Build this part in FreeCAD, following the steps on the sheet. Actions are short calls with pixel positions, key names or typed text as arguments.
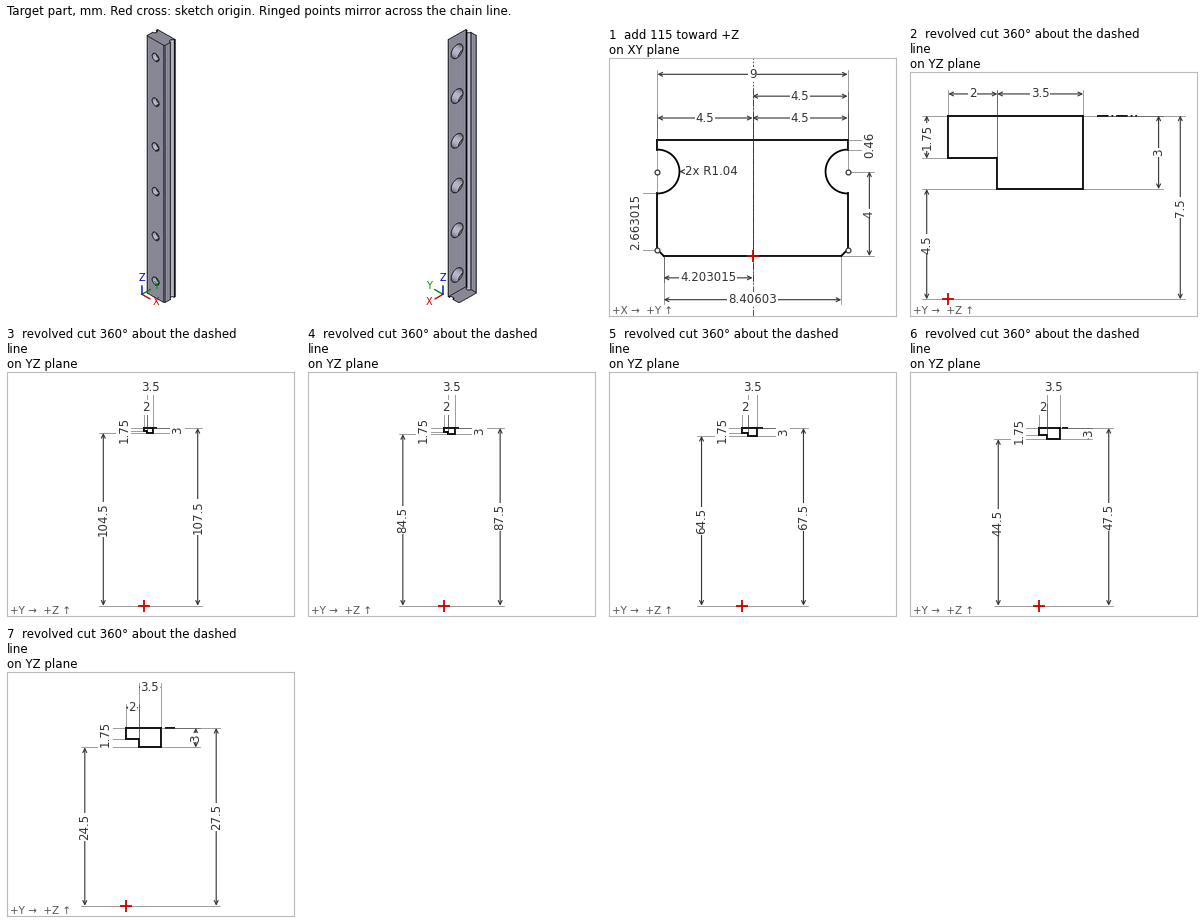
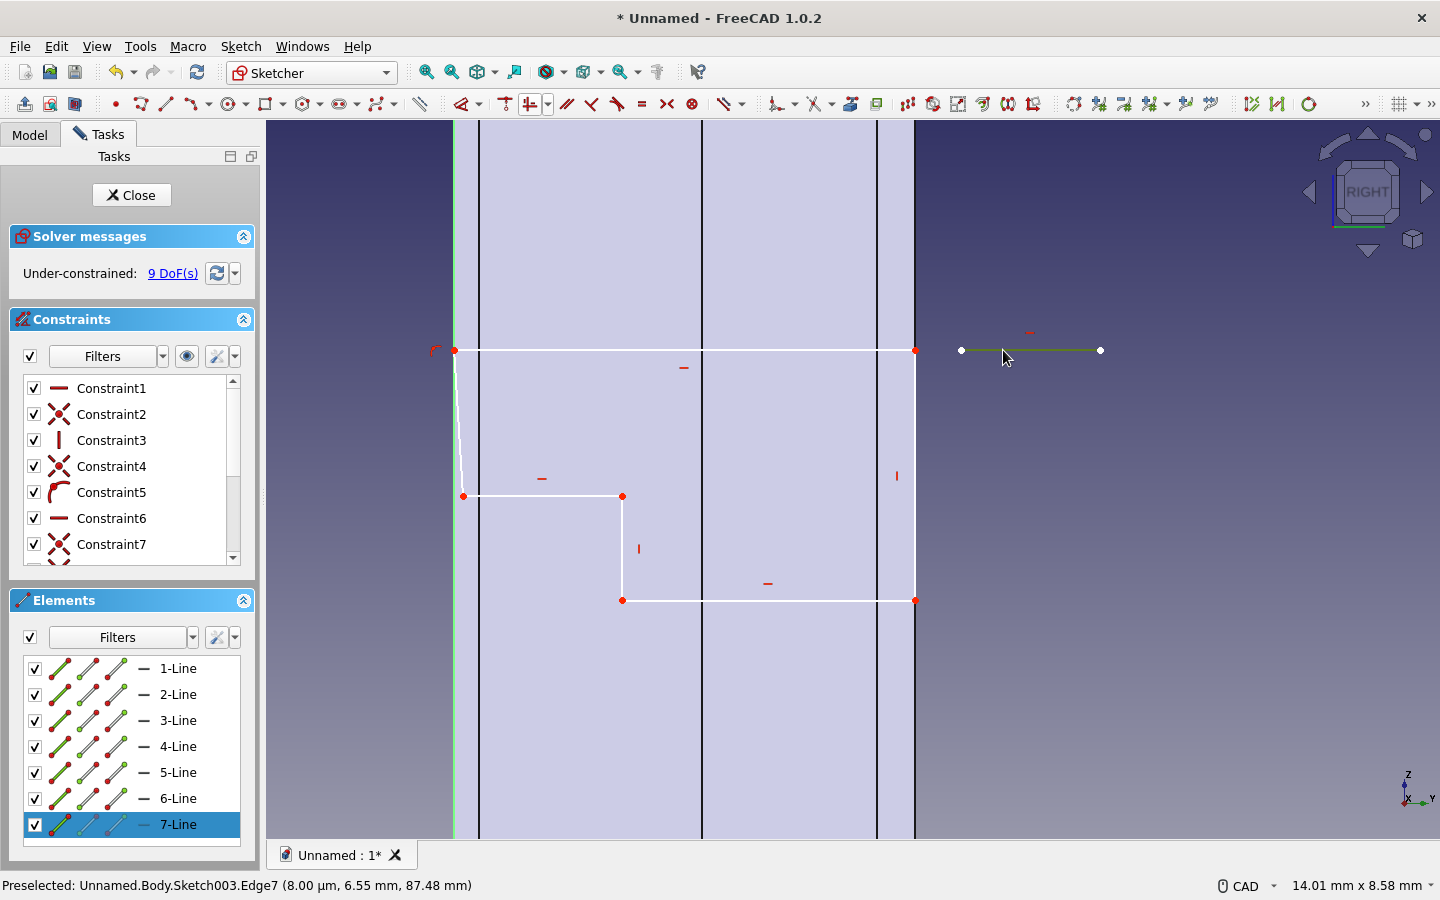
key(g)
key(n)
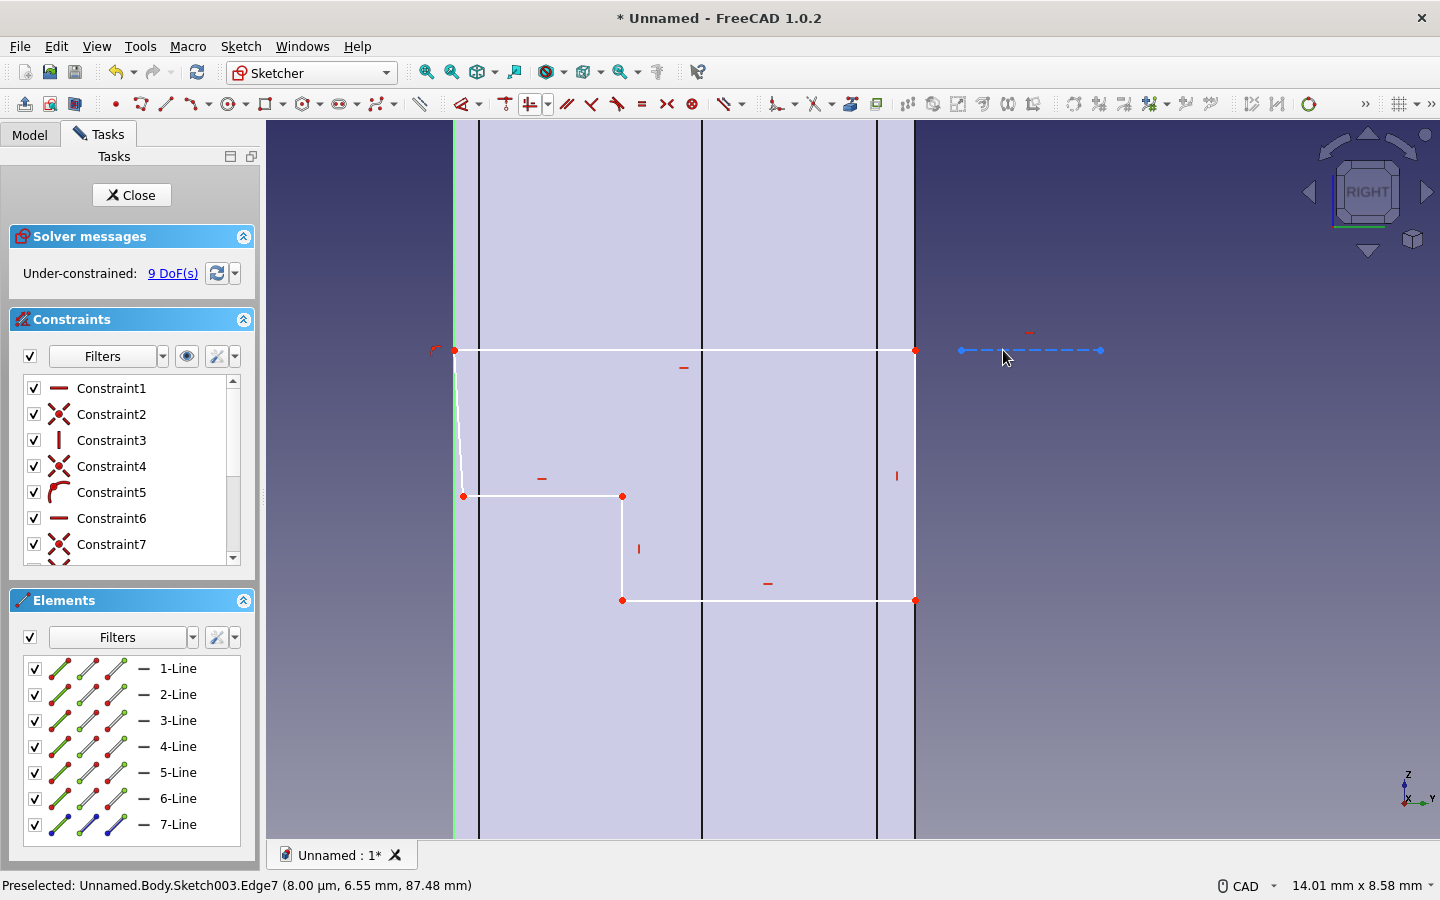
click(457, 394)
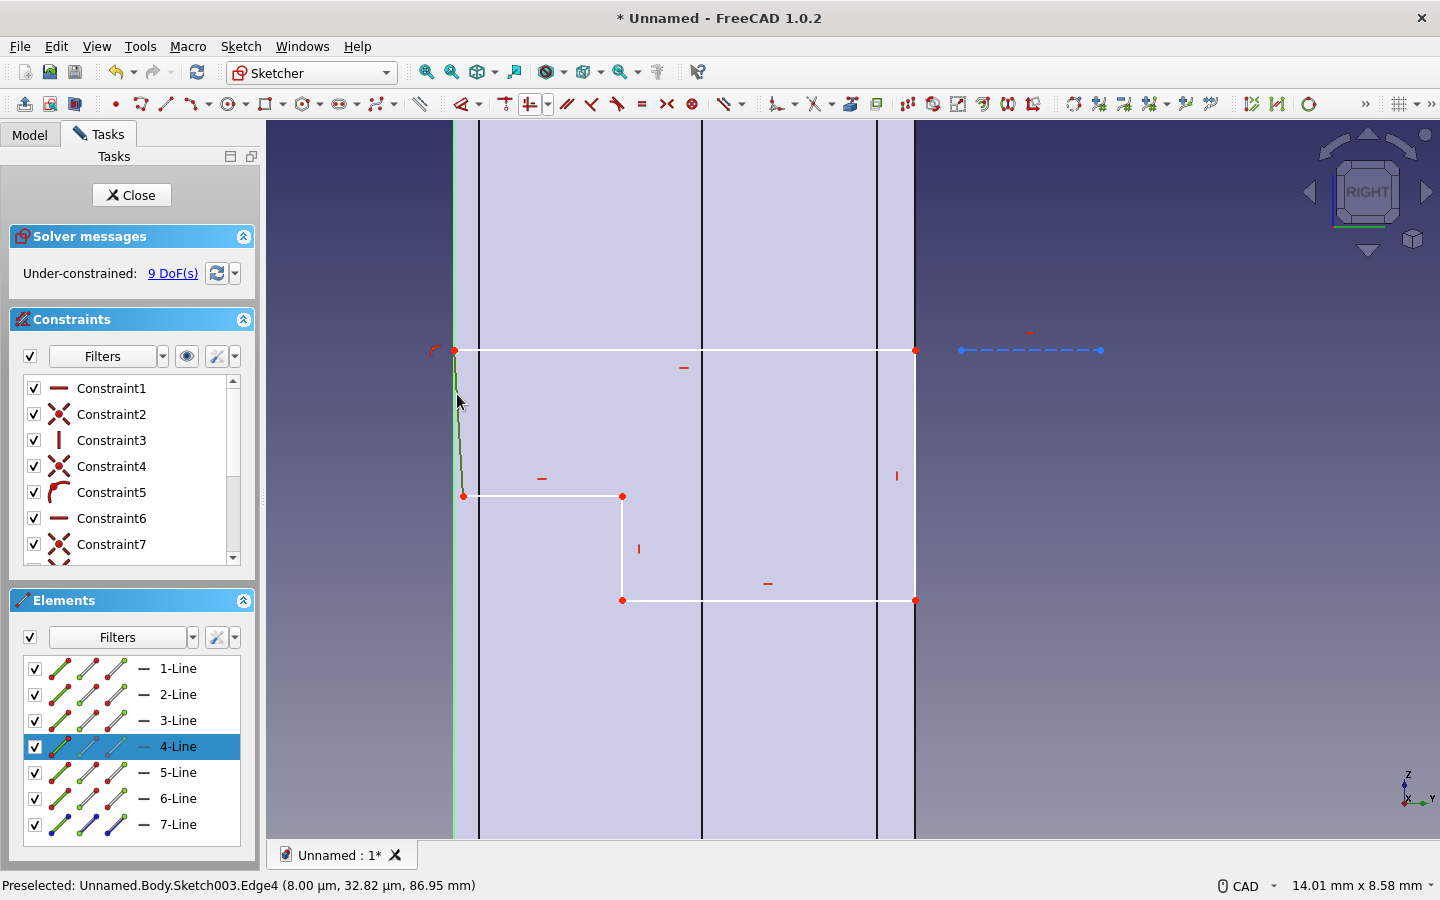
key(v)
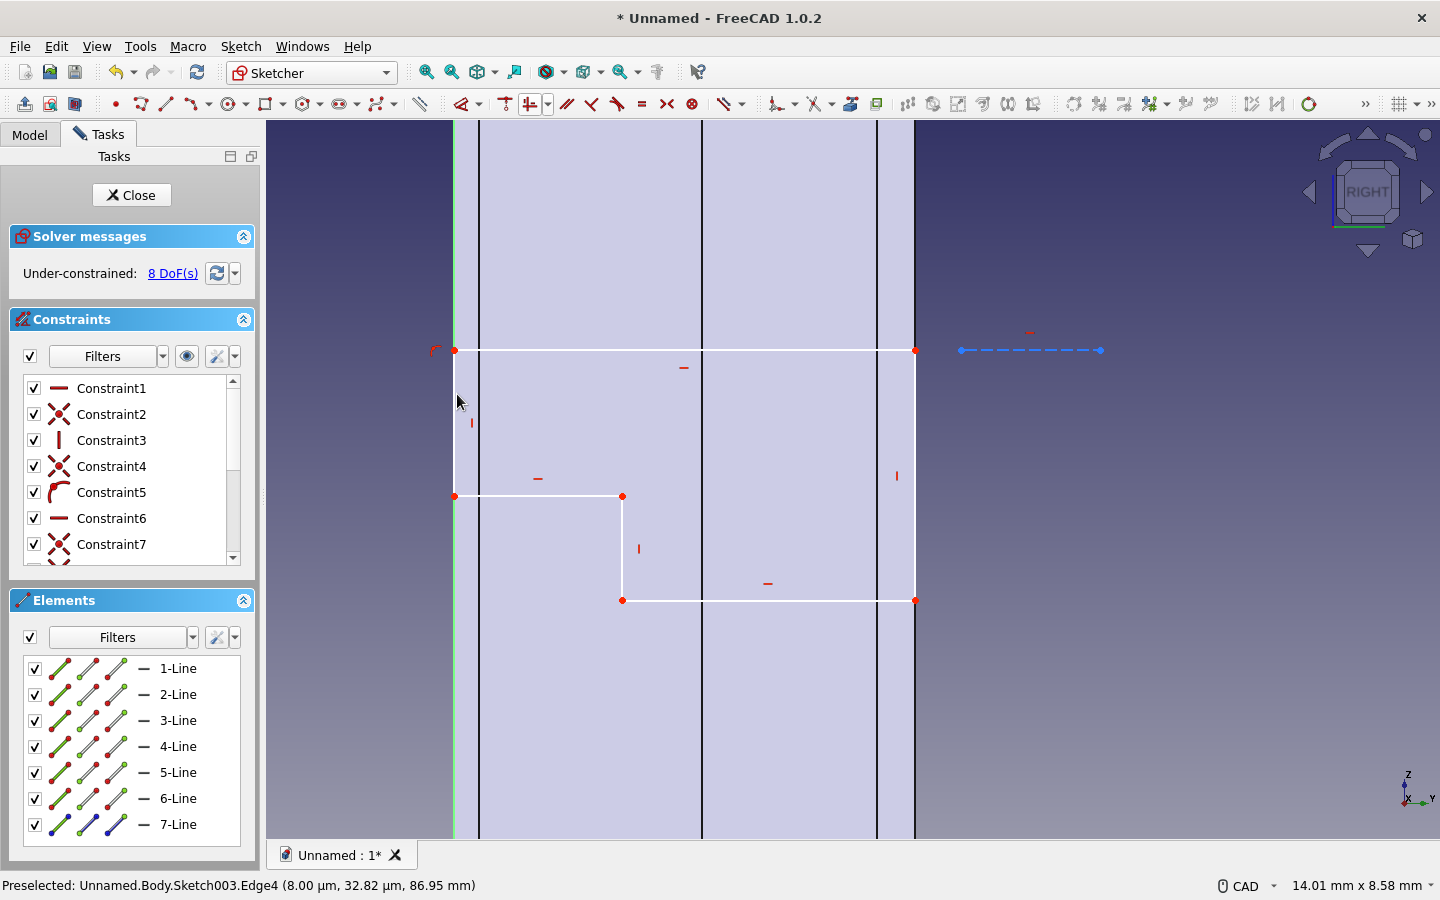
key(d)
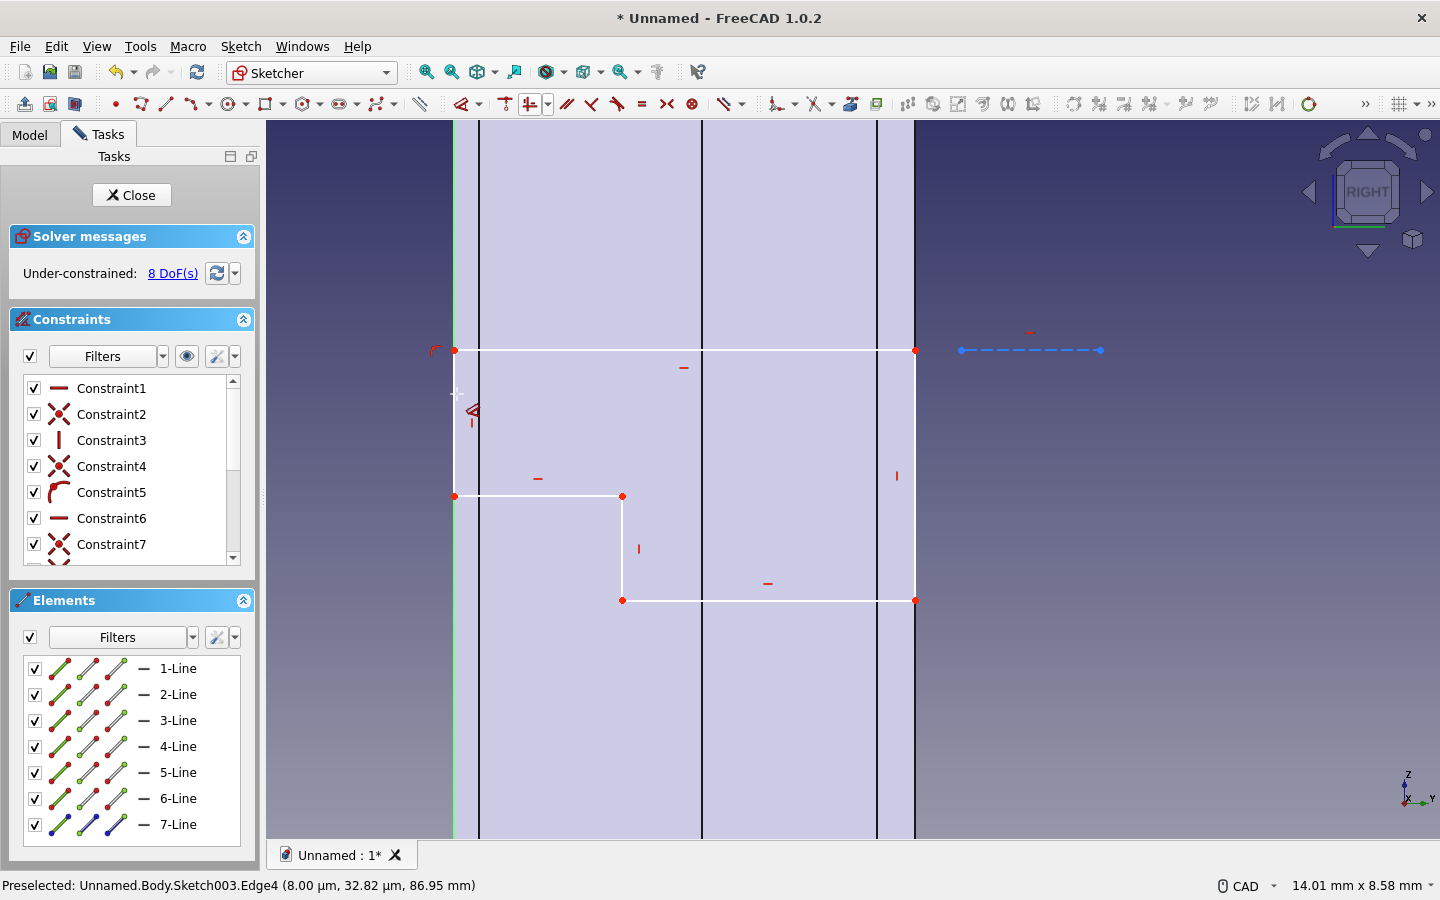
click(915, 526)
click(949, 475)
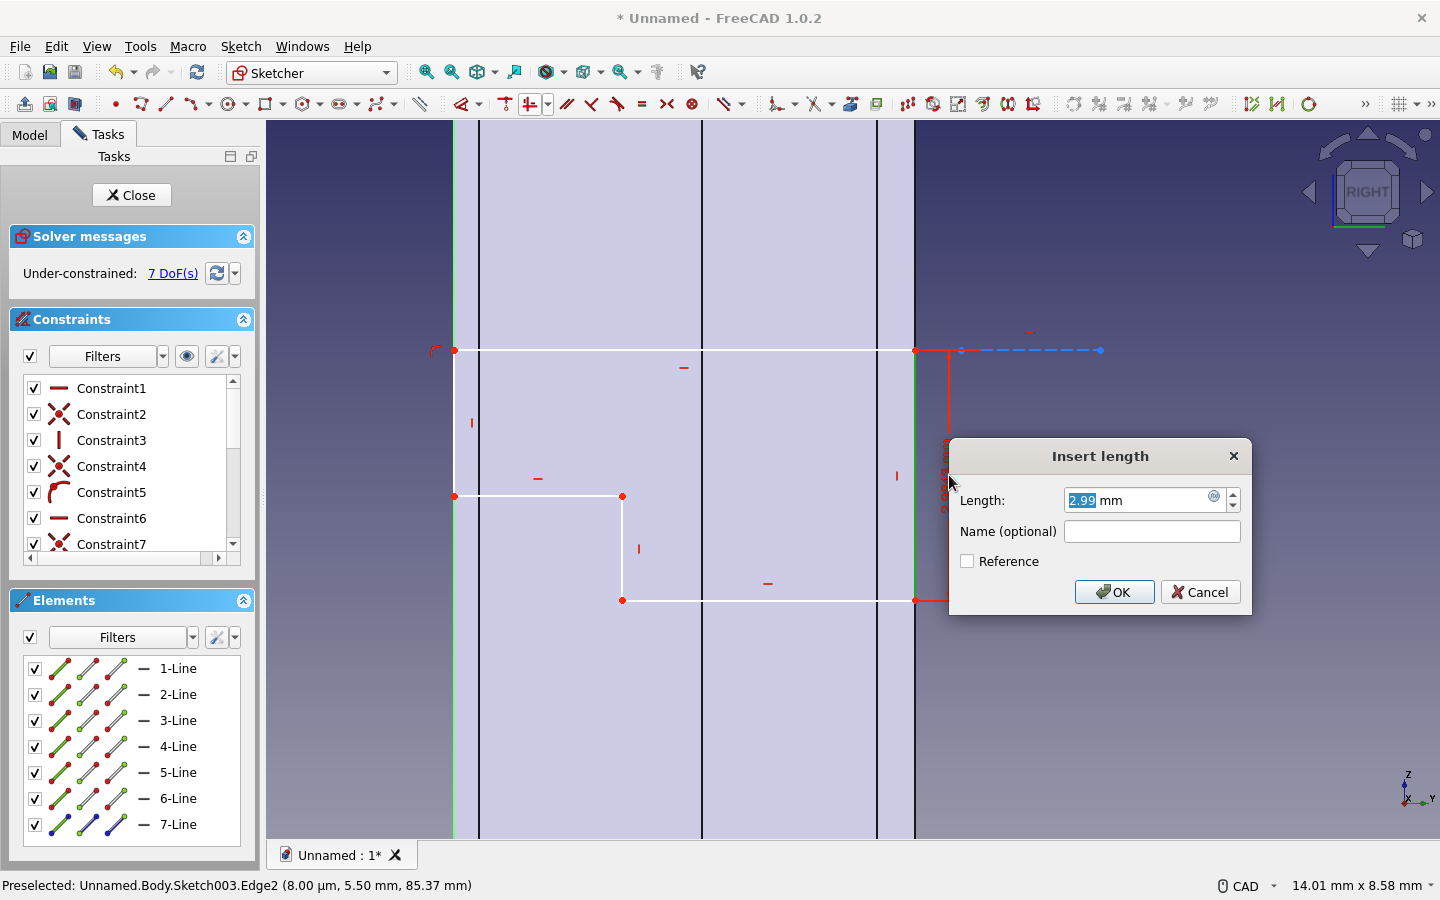
text(3)
key(Return)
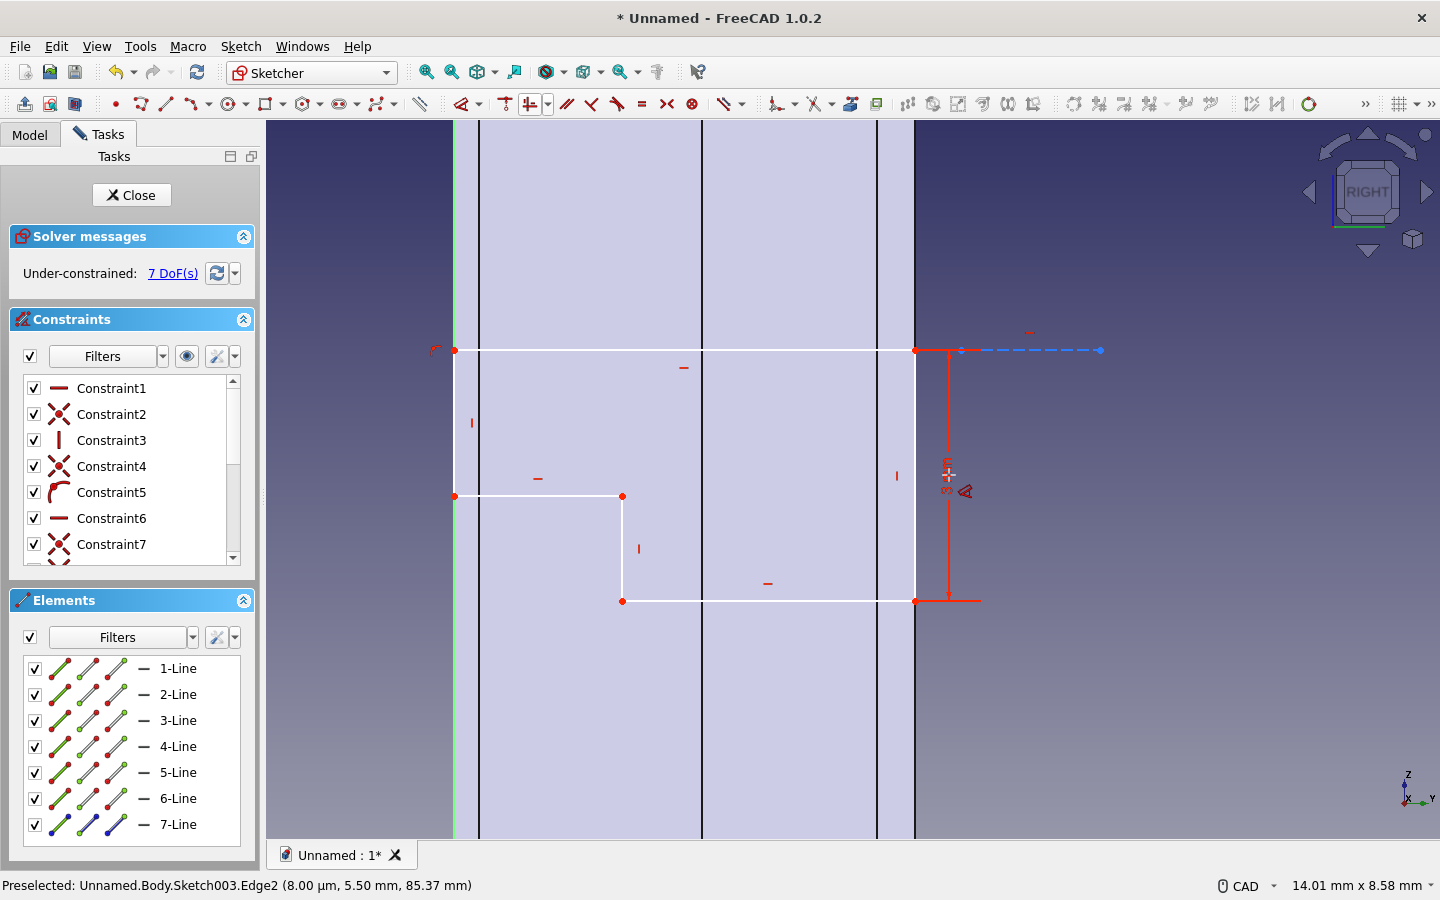
click(504, 496)
click(538, 530)